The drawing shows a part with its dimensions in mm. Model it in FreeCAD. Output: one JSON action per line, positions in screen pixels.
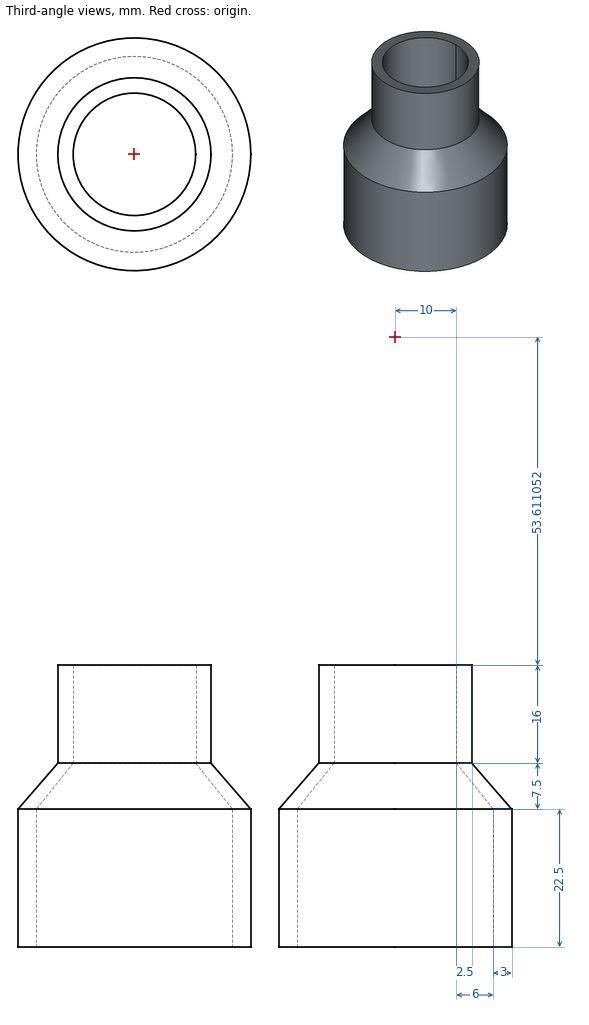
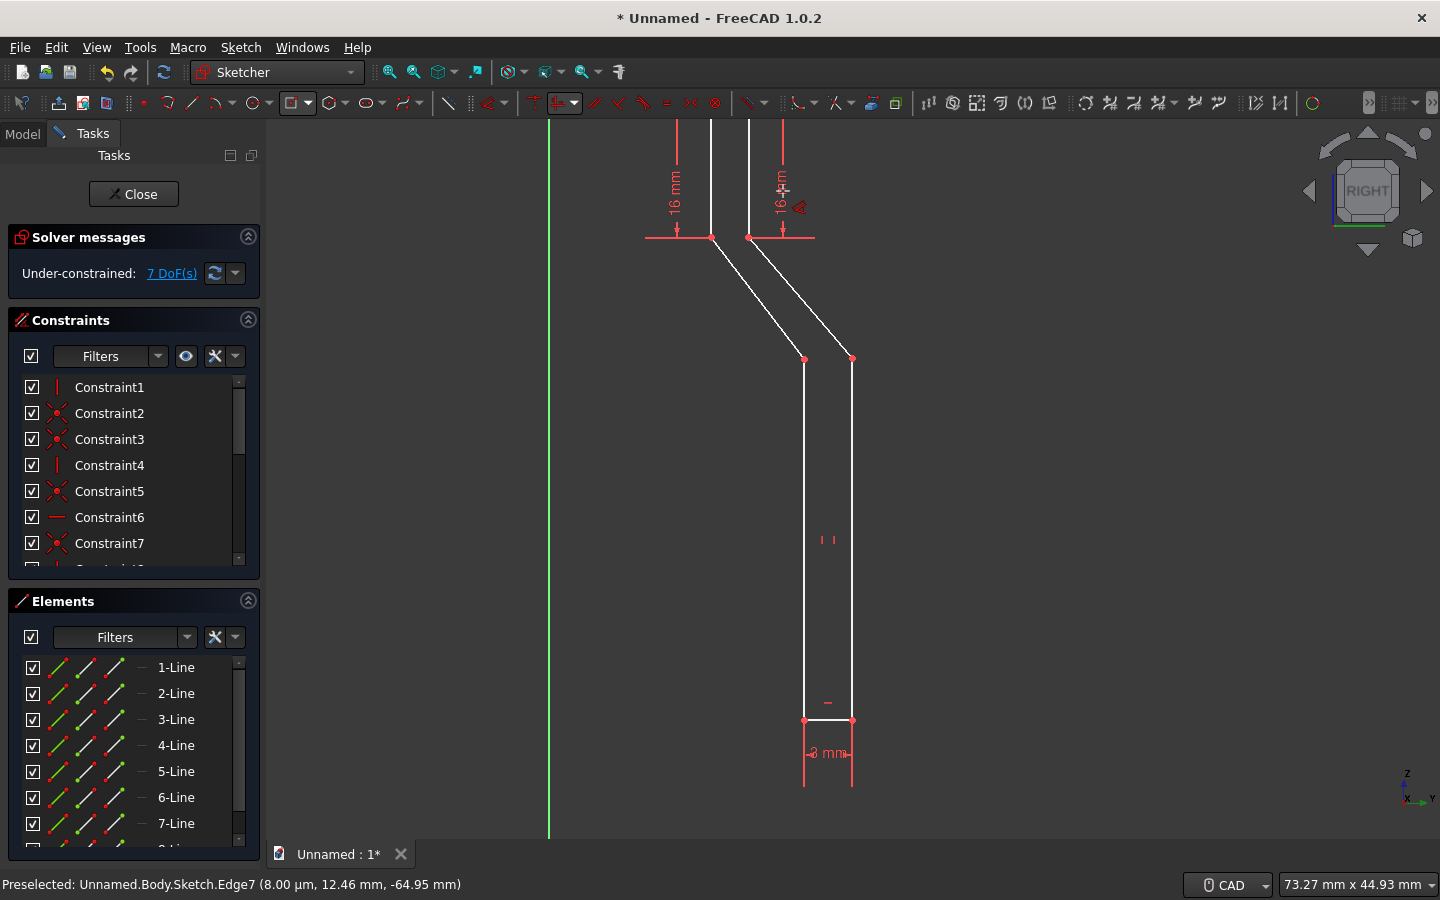
{"action": "left_click", "coordinate": [739, 274]}
{"action": "left_click", "coordinate": [758, 393]}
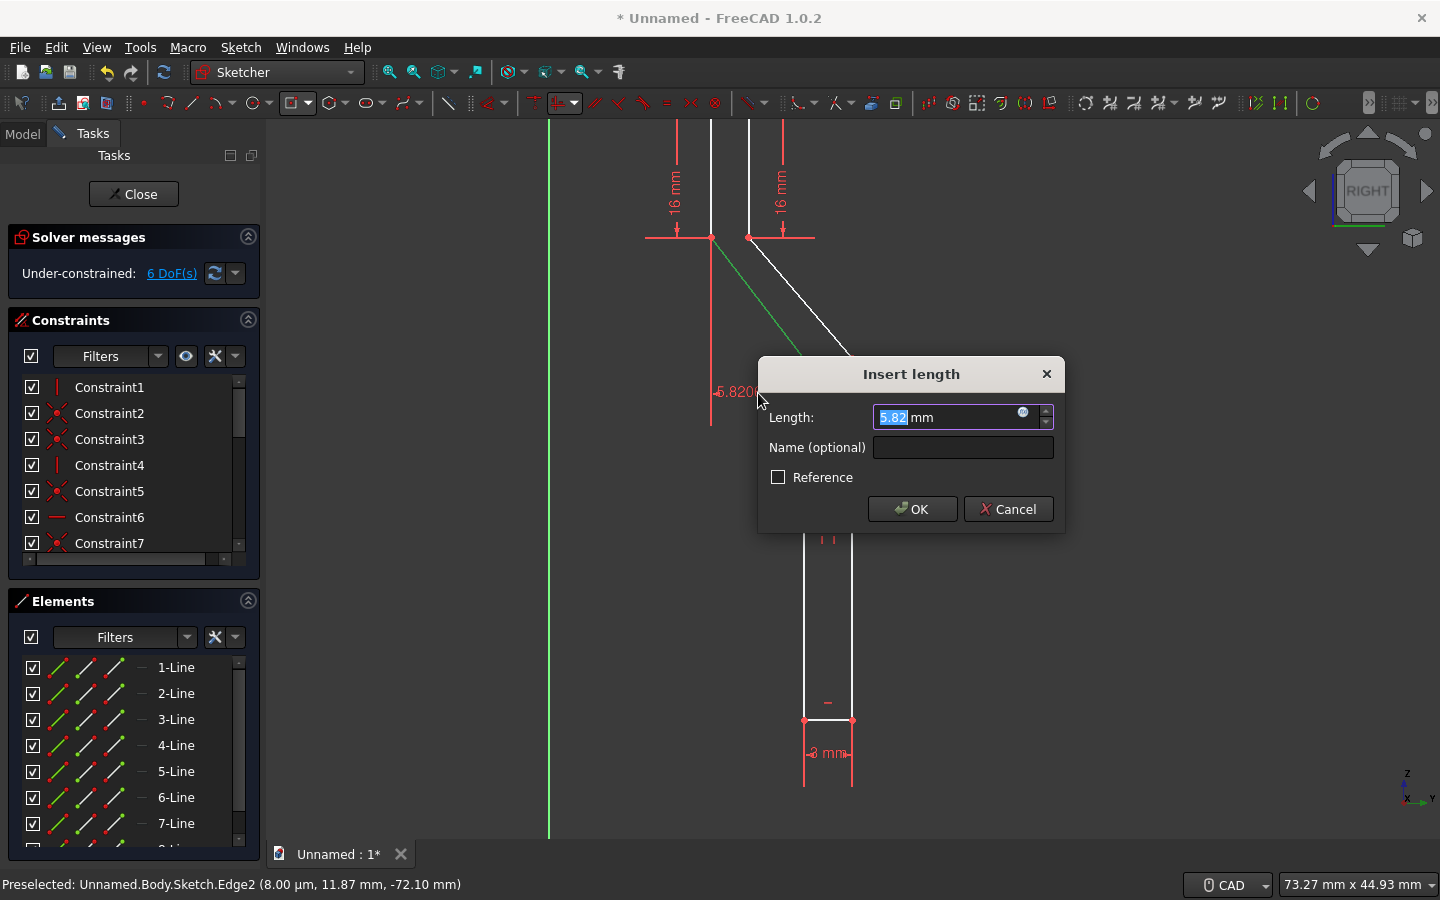
{"action": "type", "text": "6"}
{"action": "key", "text": "Return"}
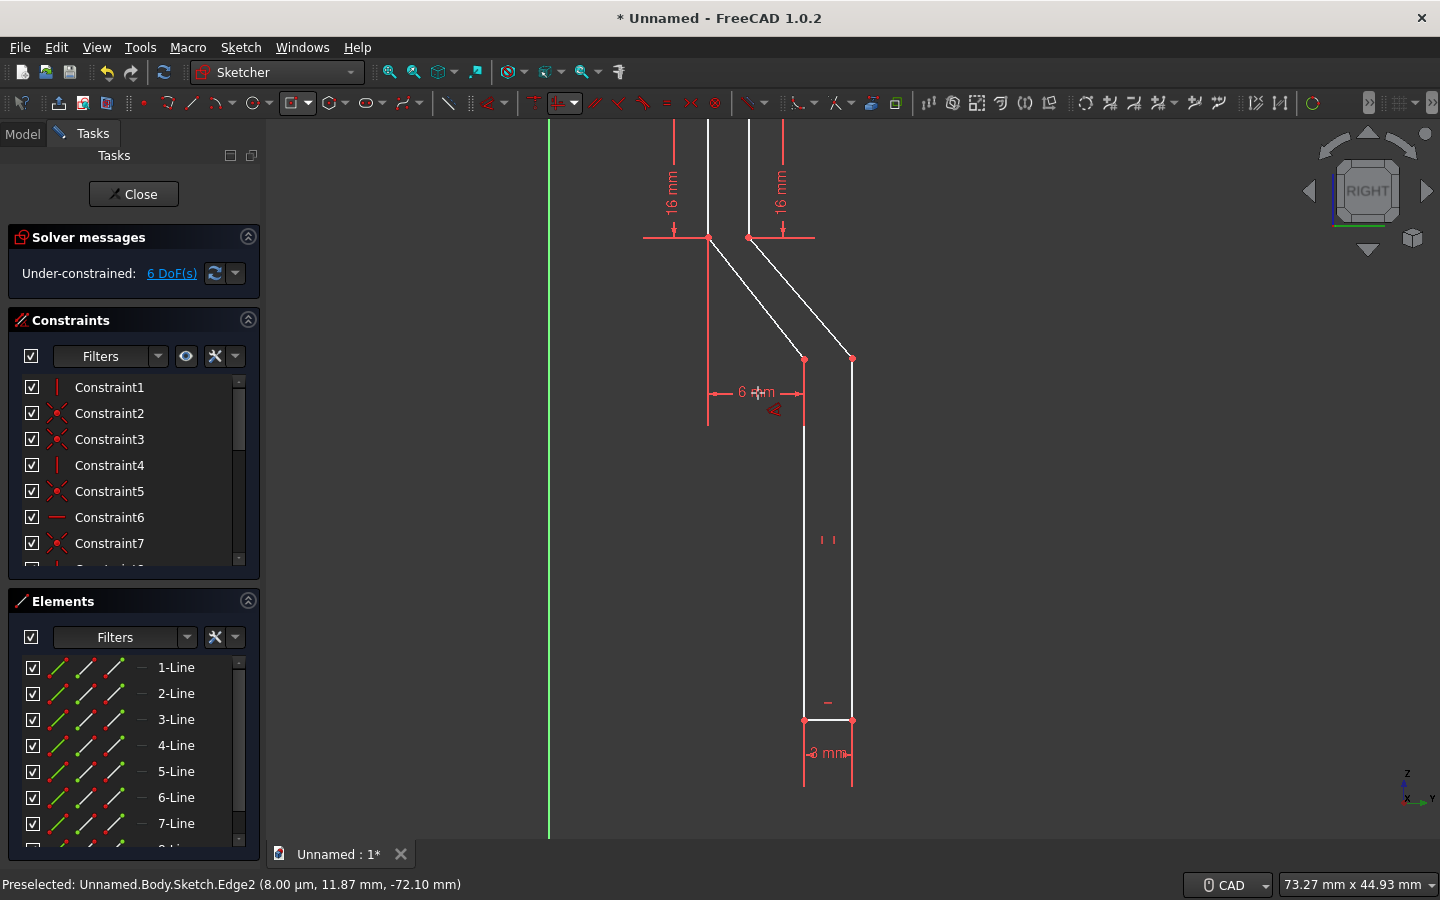
{"action": "scroll", "coordinate": [820, 721], "scroll_direction": "down", "scroll_amount": 6}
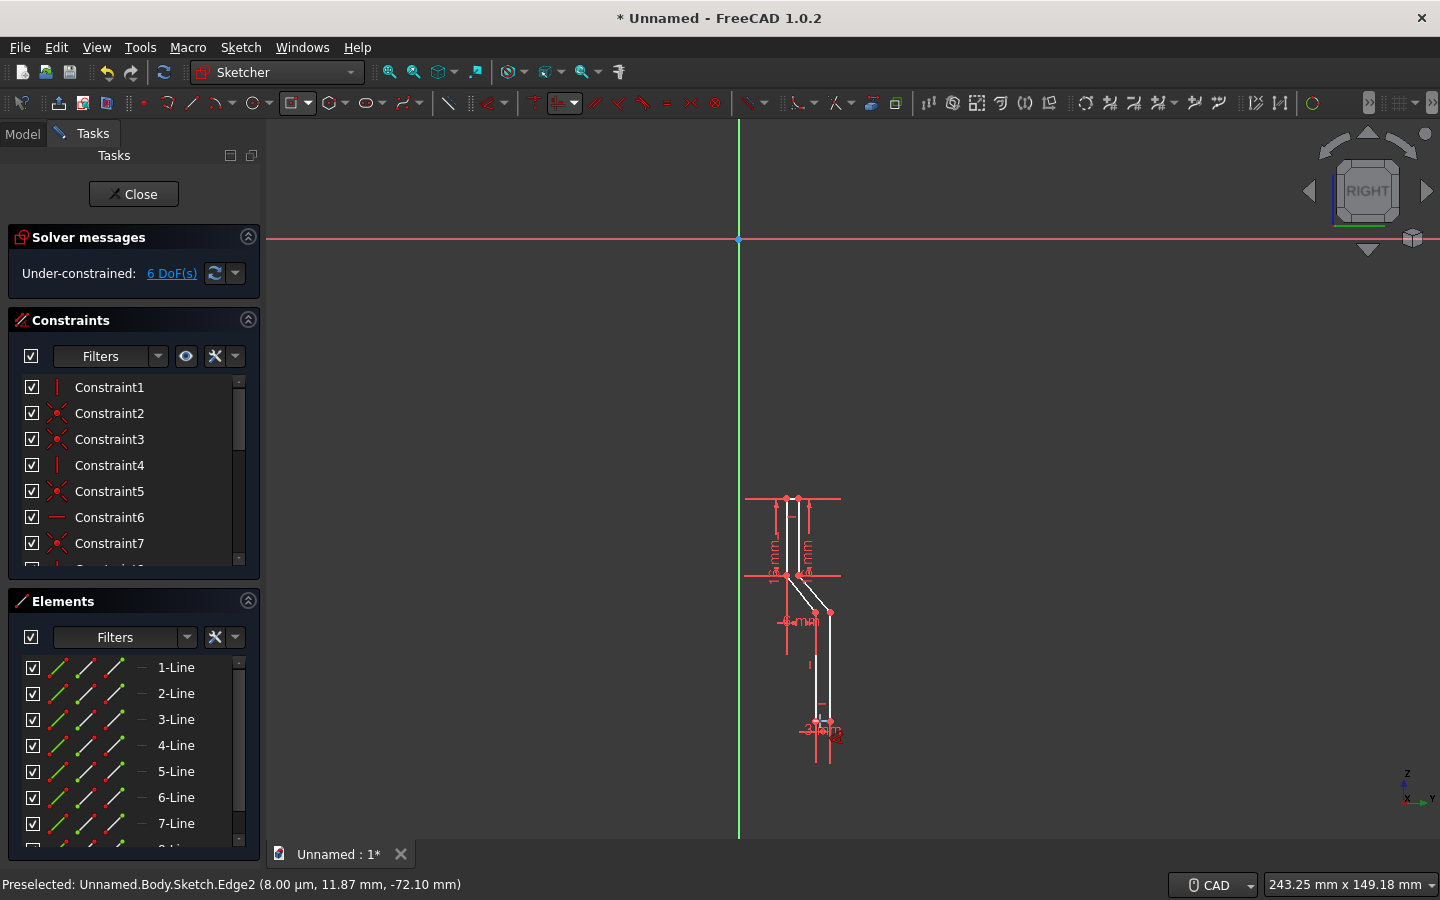
{"action": "scroll", "coordinate": [795, 499], "scroll_direction": "up", "scroll_amount": 7}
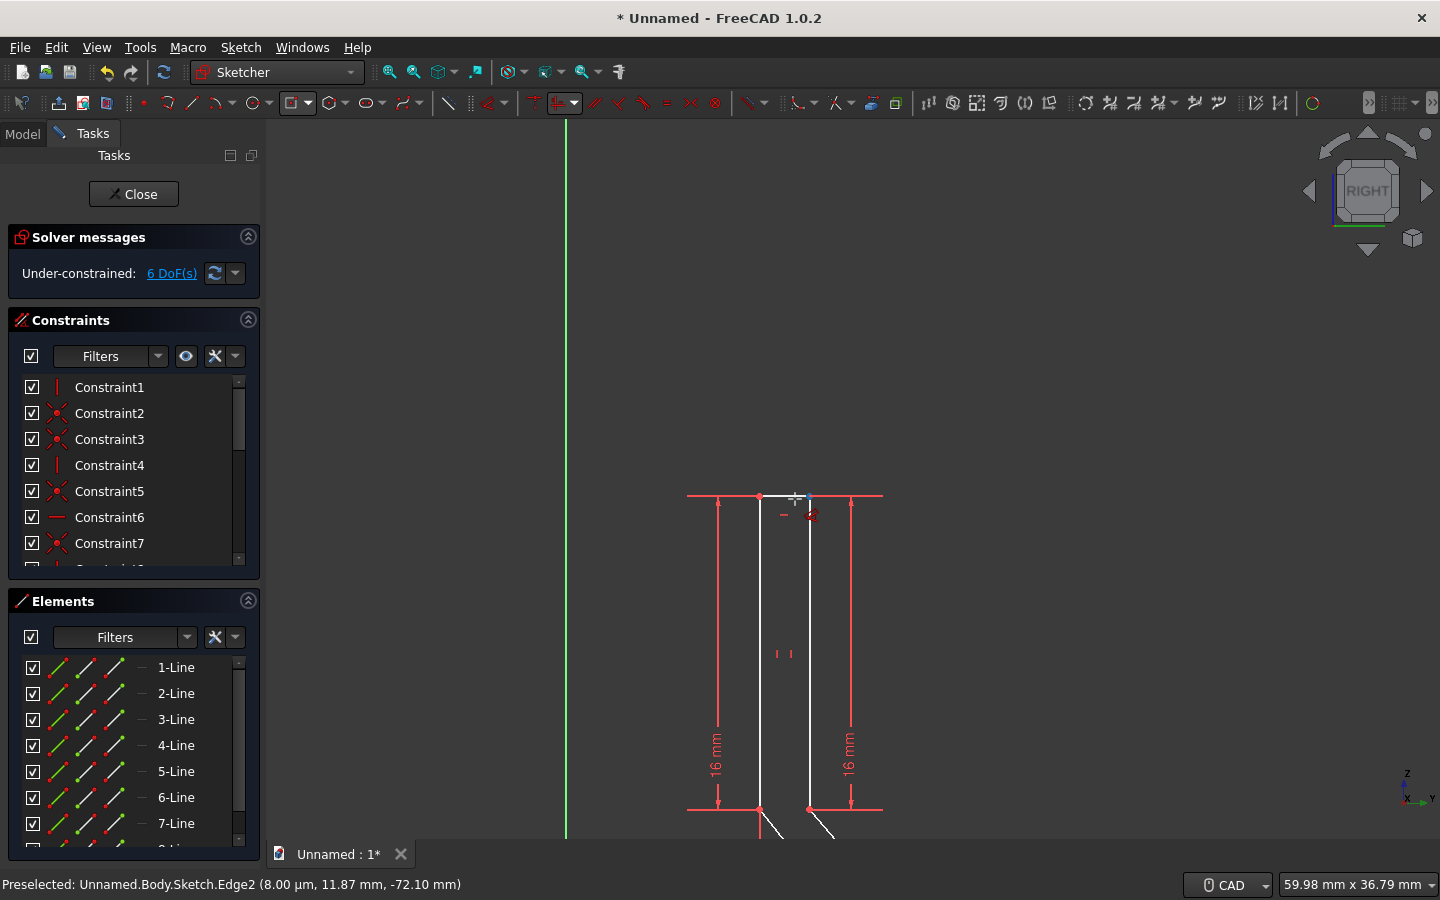
{"action": "left_click", "coordinate": [795, 496]}
{"action": "left_click", "coordinate": [785, 530]}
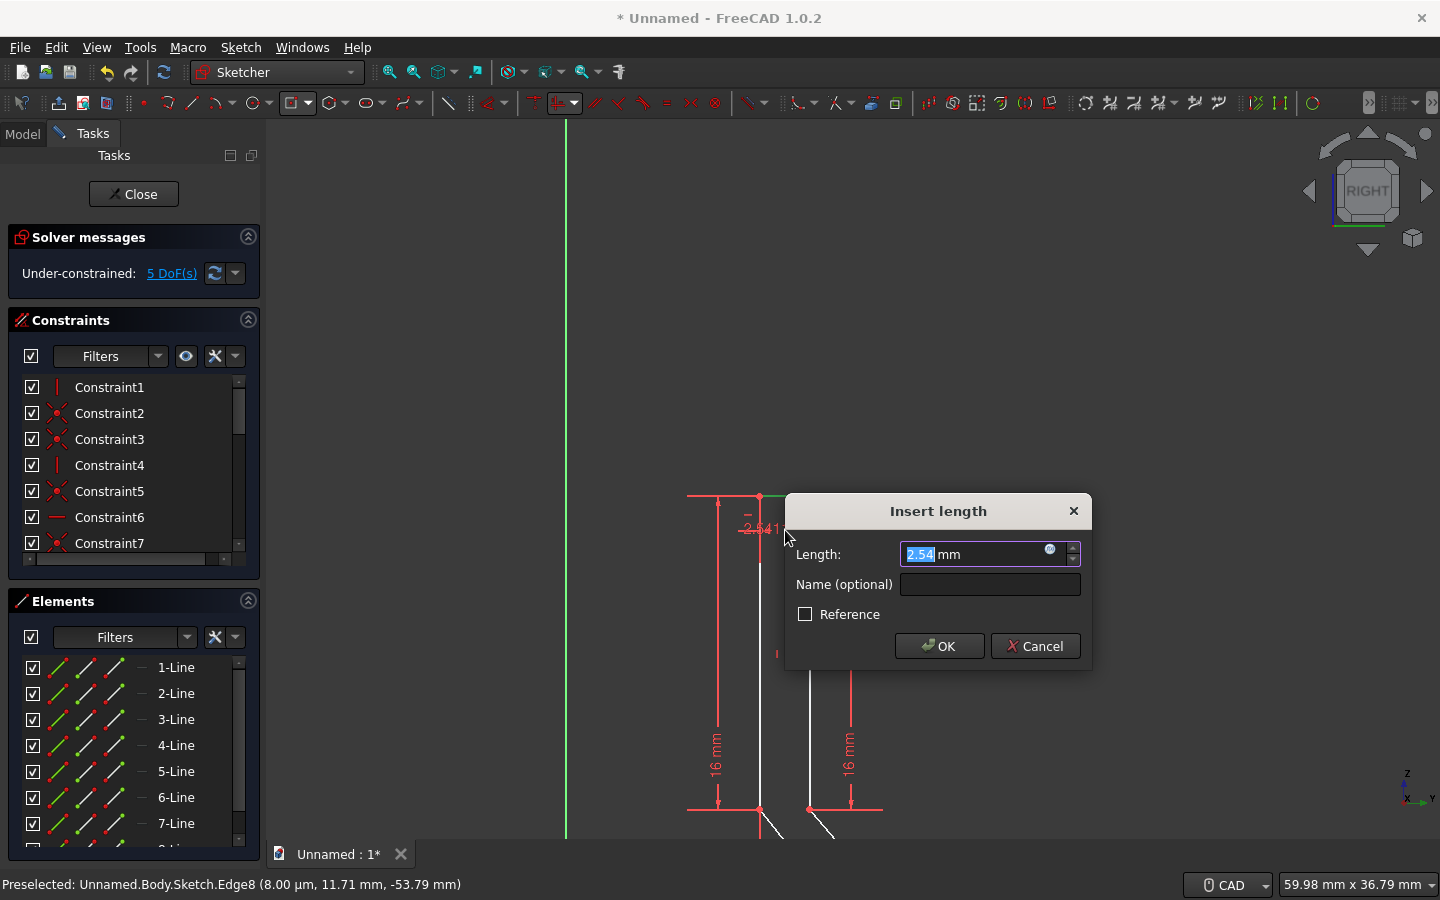
{"action": "type", "text": "2.5"}
{"action": "key", "text": "Return"}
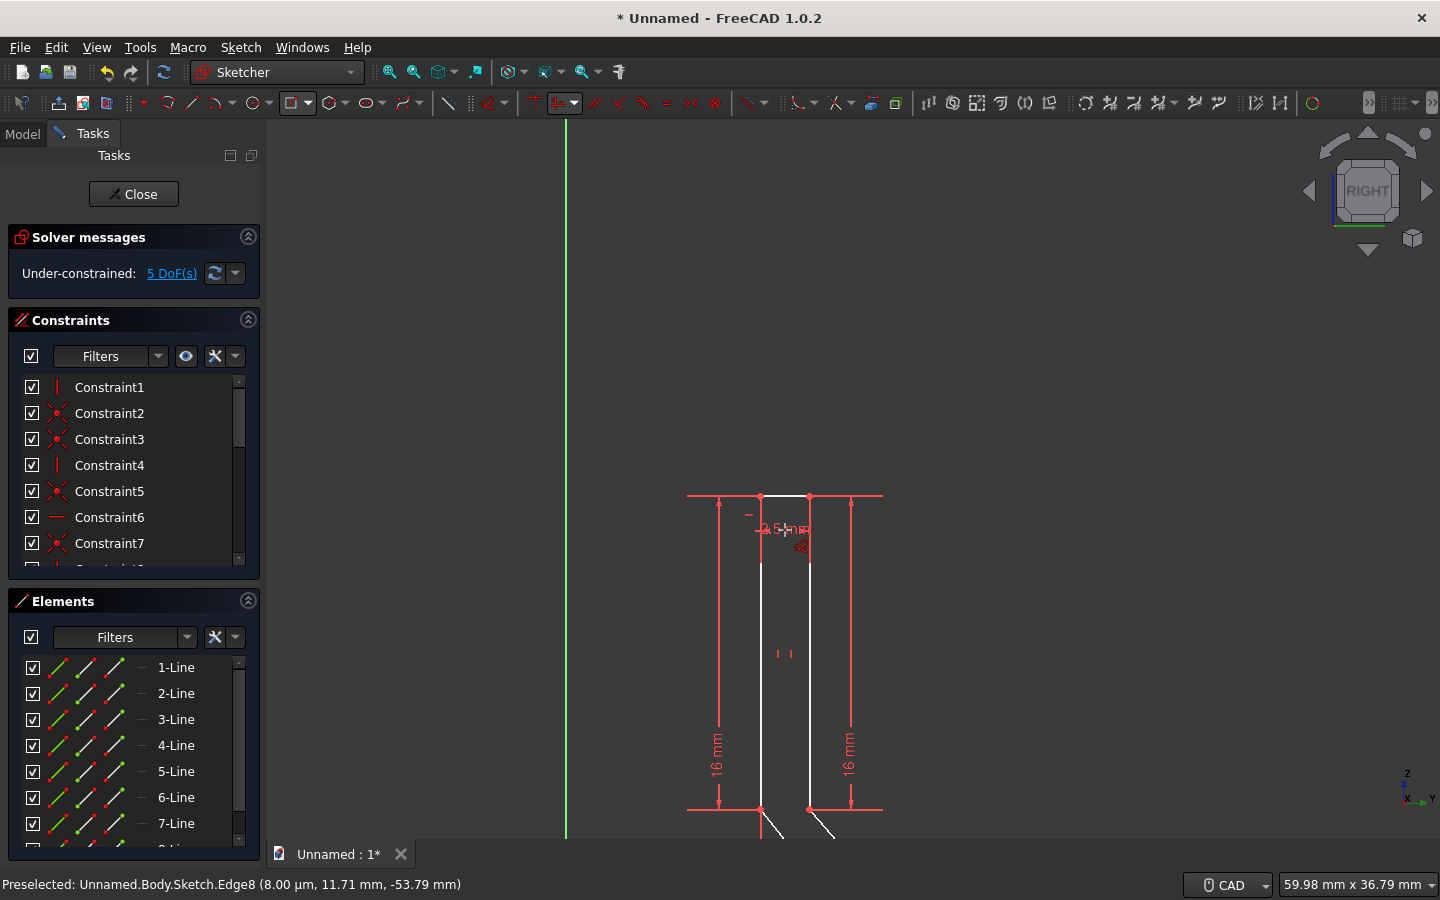
{"action": "scroll", "coordinate": [795, 499], "scroll_direction": "down", "scroll_amount": 7}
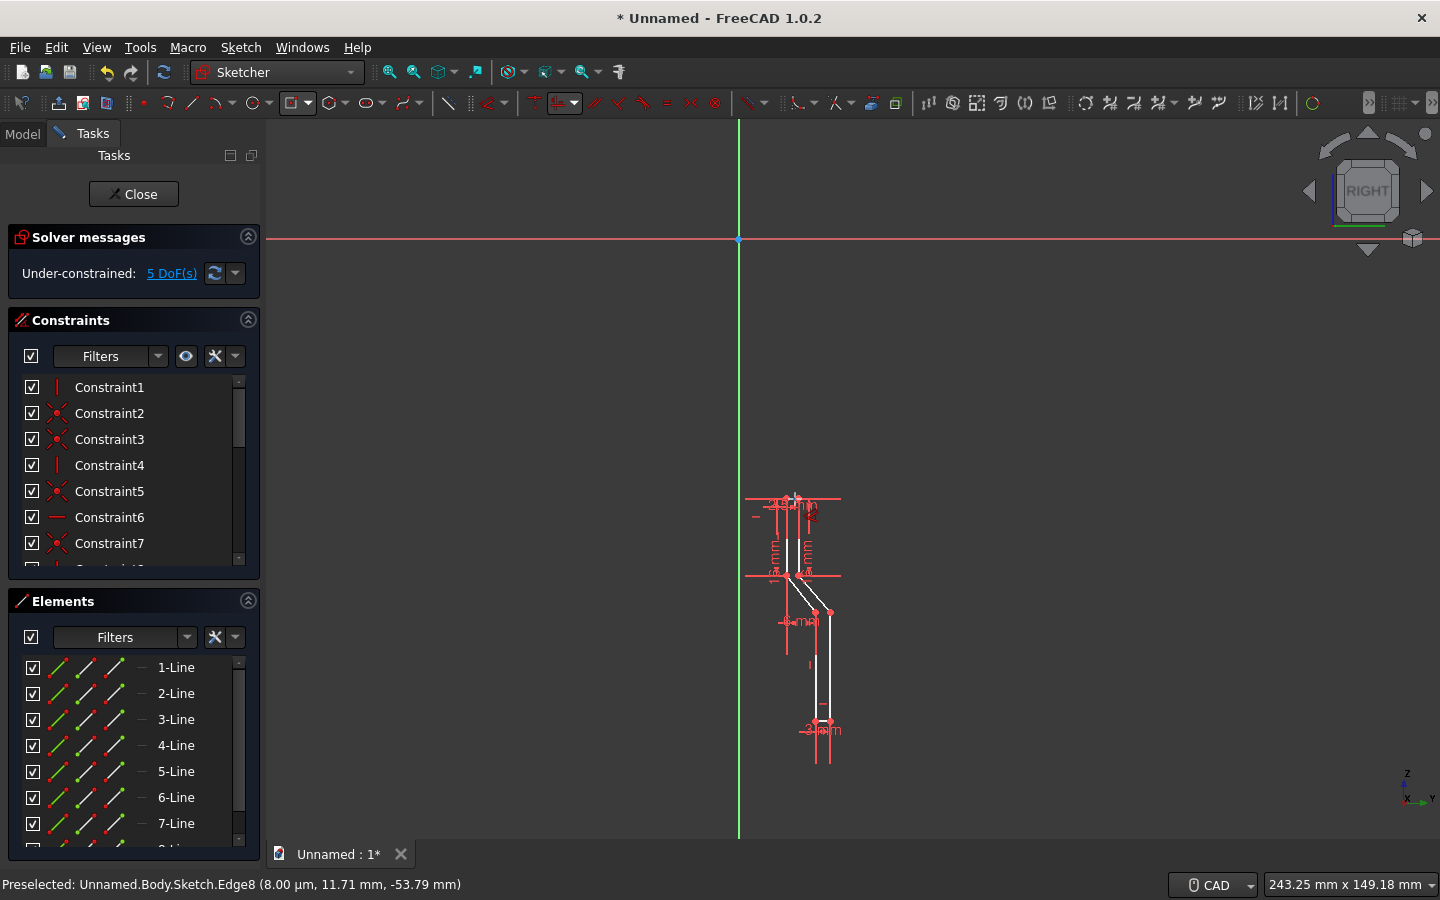
{"action": "left_click", "coordinate": [787, 499]}
{"action": "left_click", "coordinate": [763, 205]}